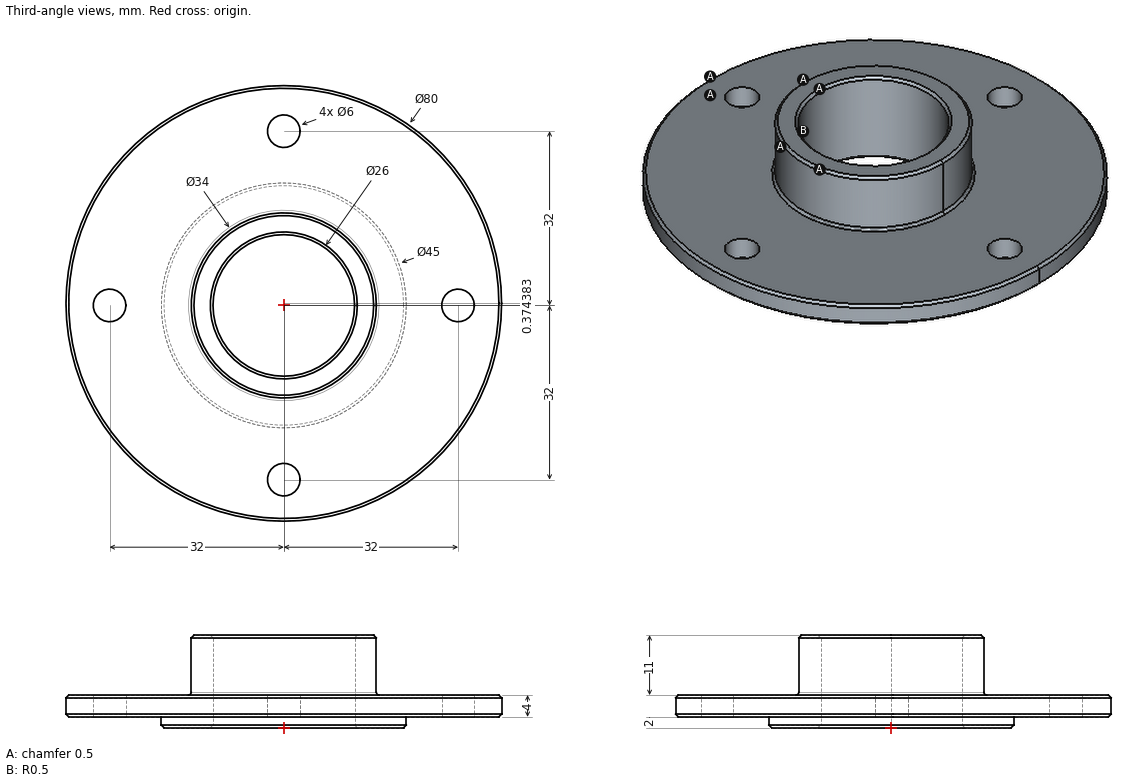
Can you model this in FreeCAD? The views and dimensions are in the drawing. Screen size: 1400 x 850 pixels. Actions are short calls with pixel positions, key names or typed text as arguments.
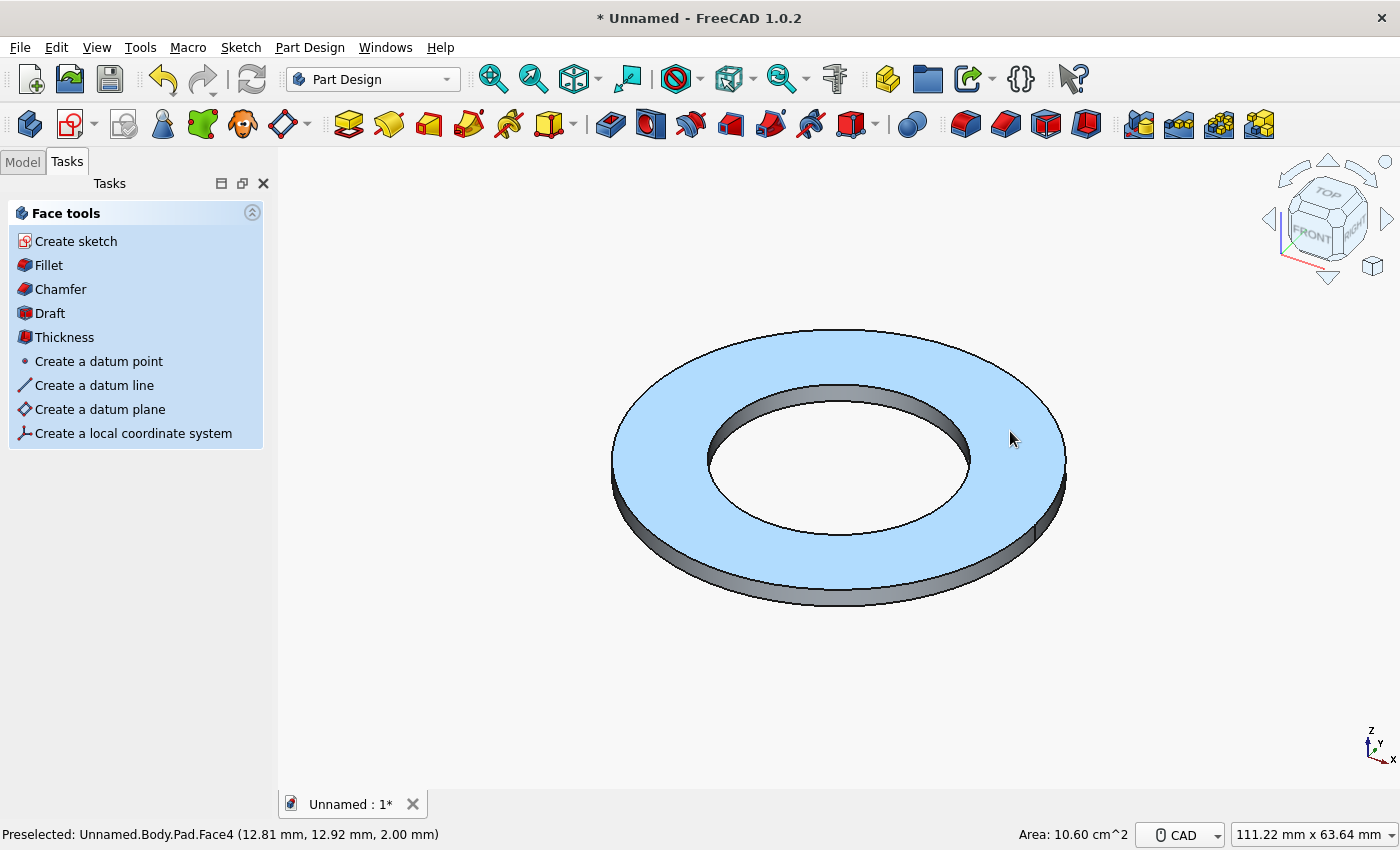
click(70, 124)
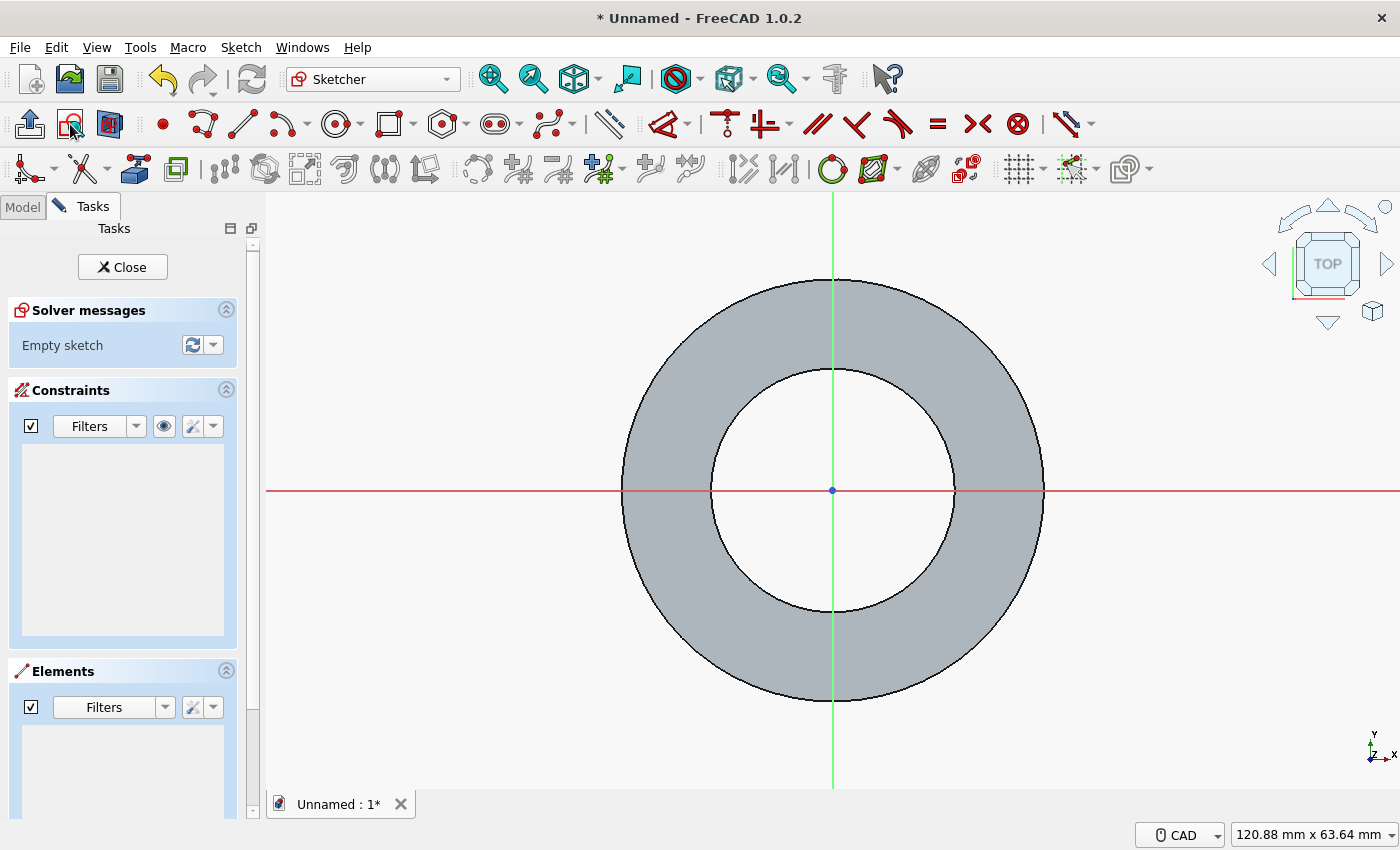
scroll(681, 495, down, 3)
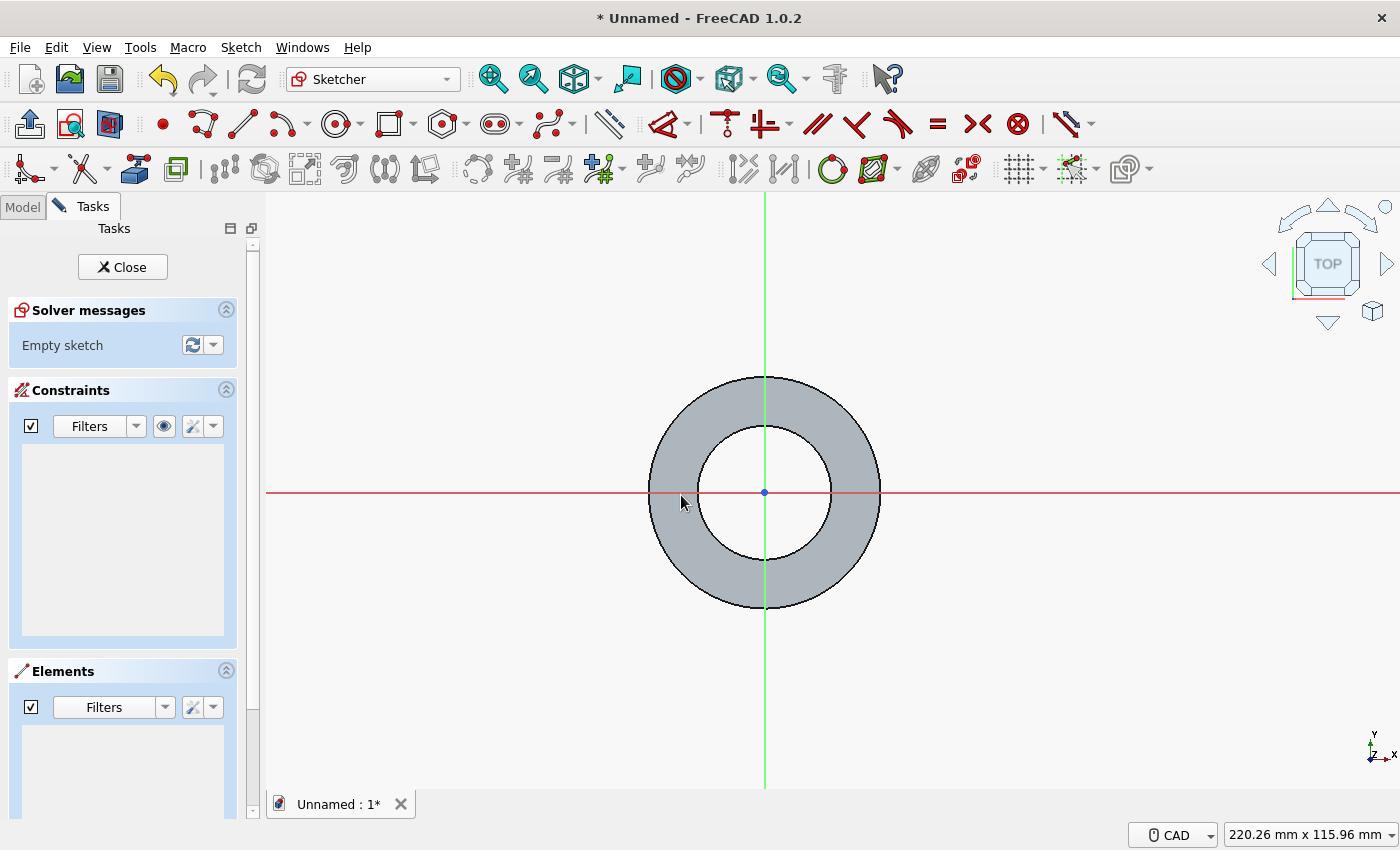
click(336, 124)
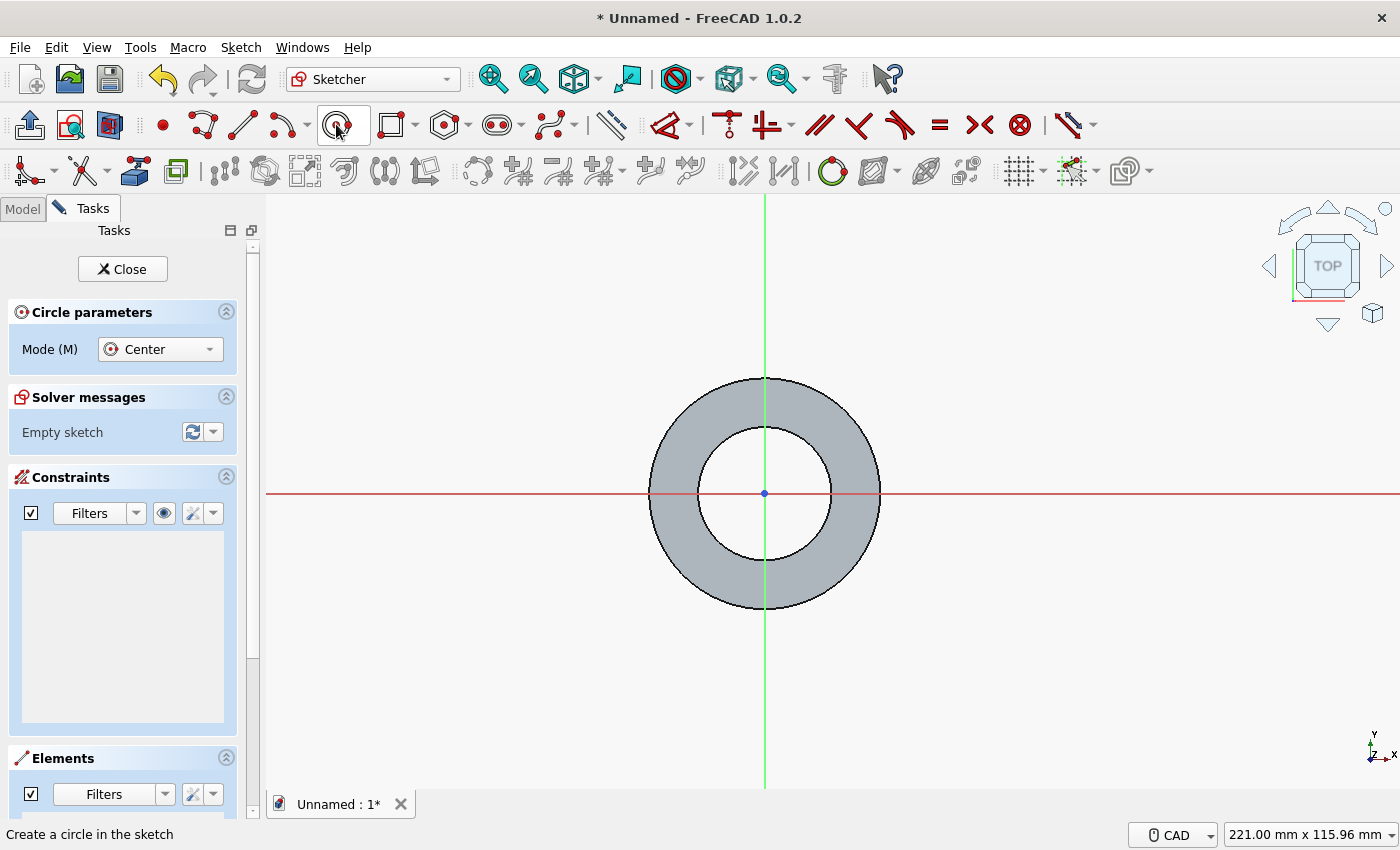
scroll(765, 492, up, 11)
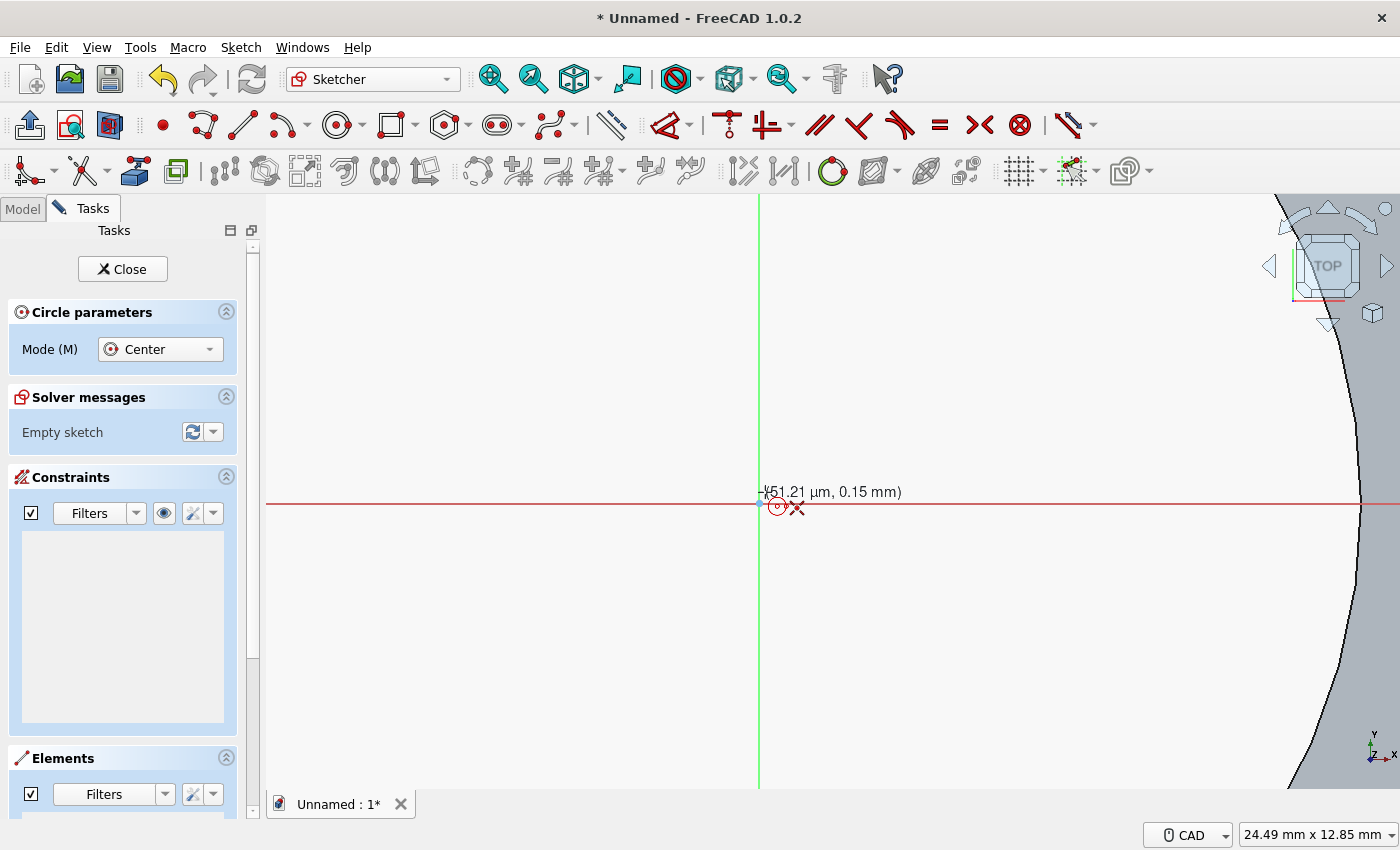
click(759, 486)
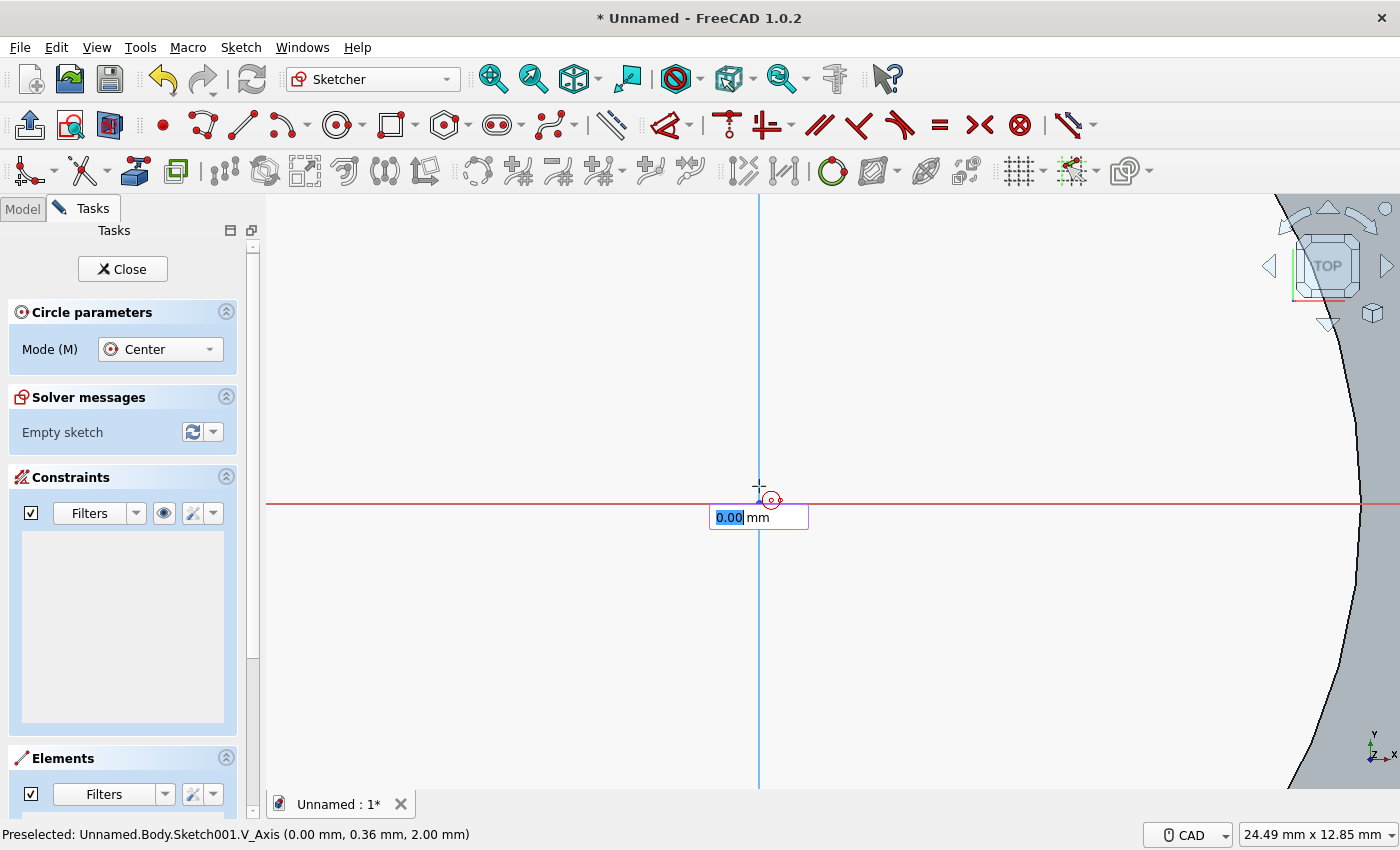
scroll(765, 492, down, 11)
move(910, 347)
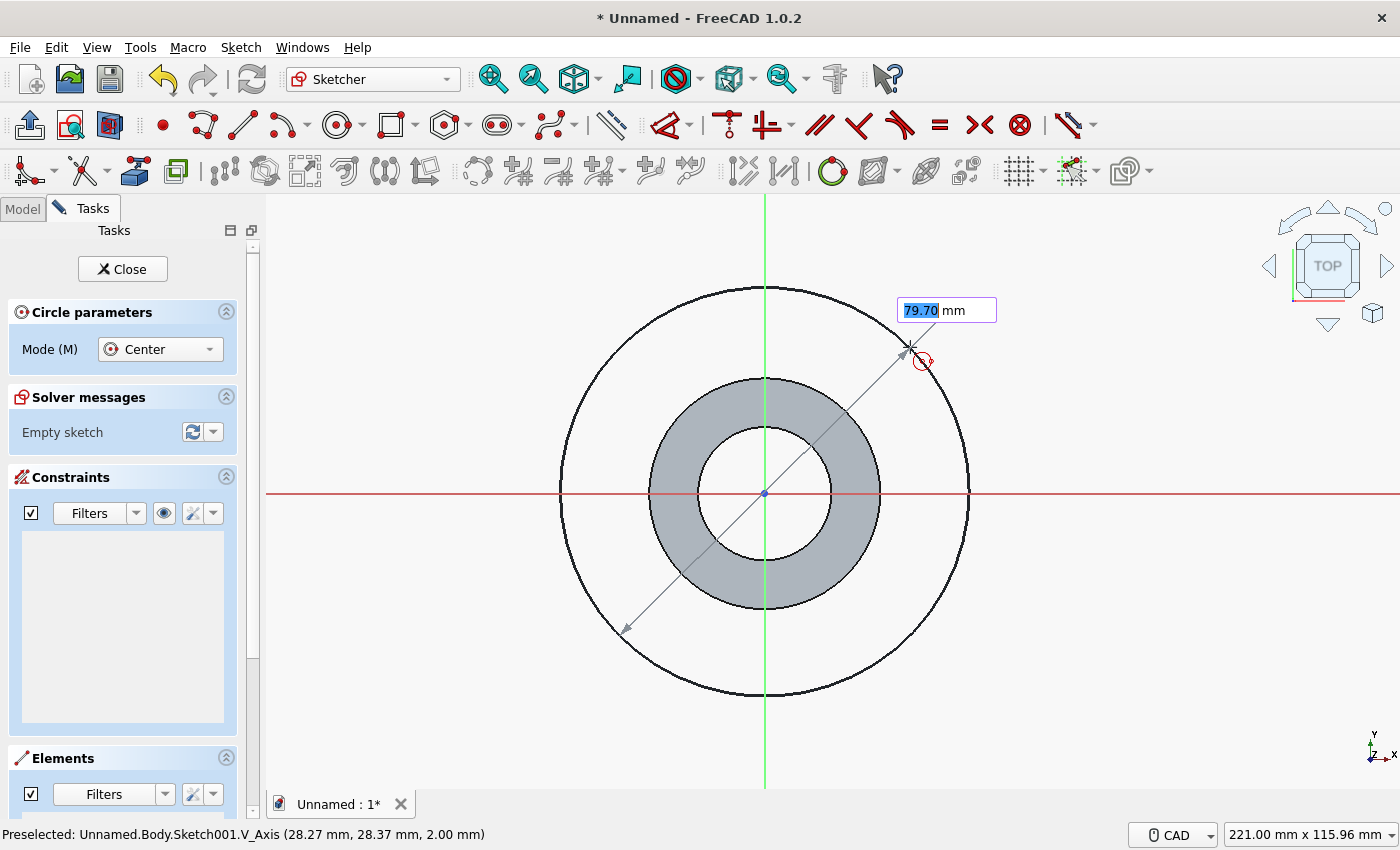
text(80)
key(Return)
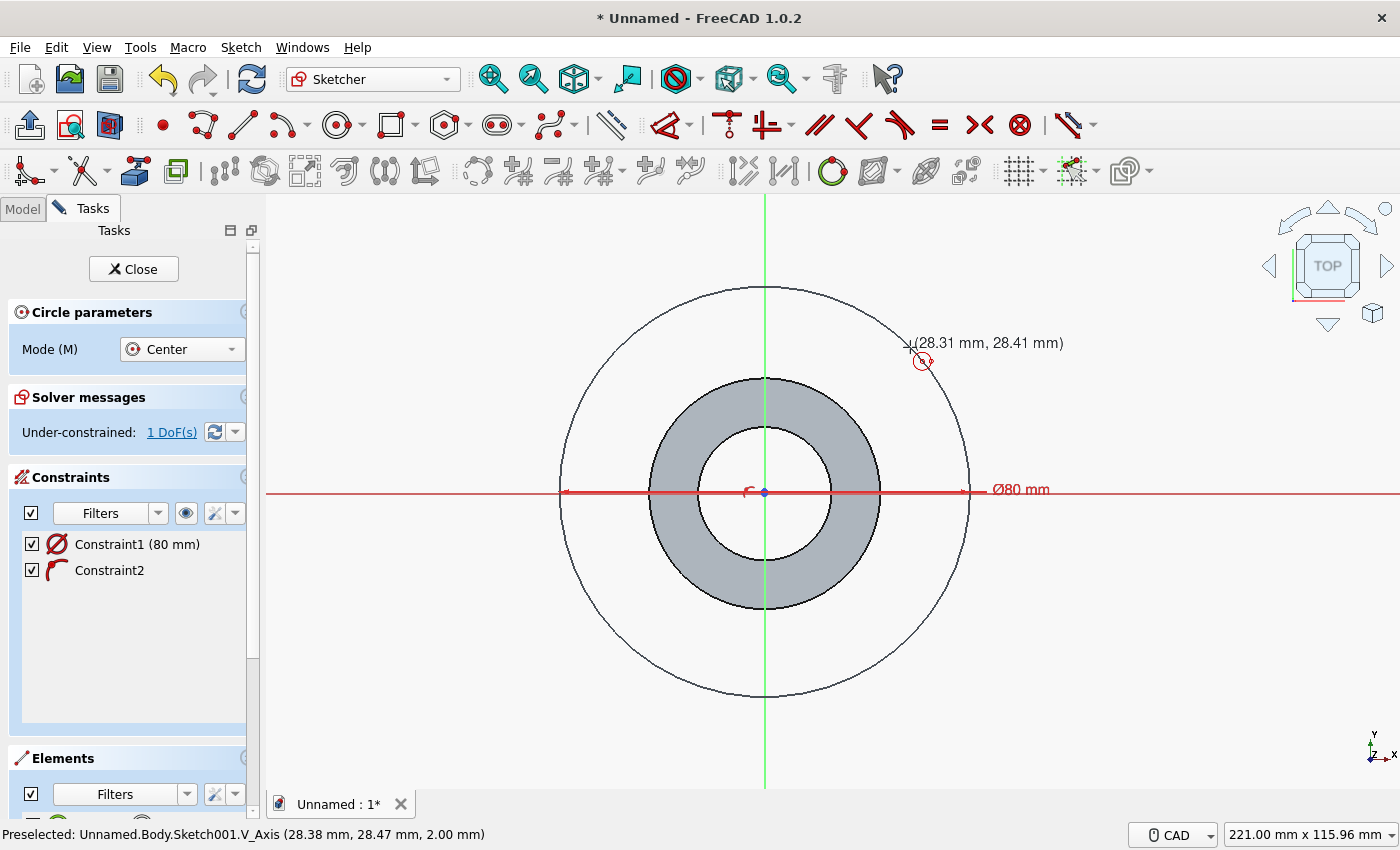
scroll(765, 494, up, 11)